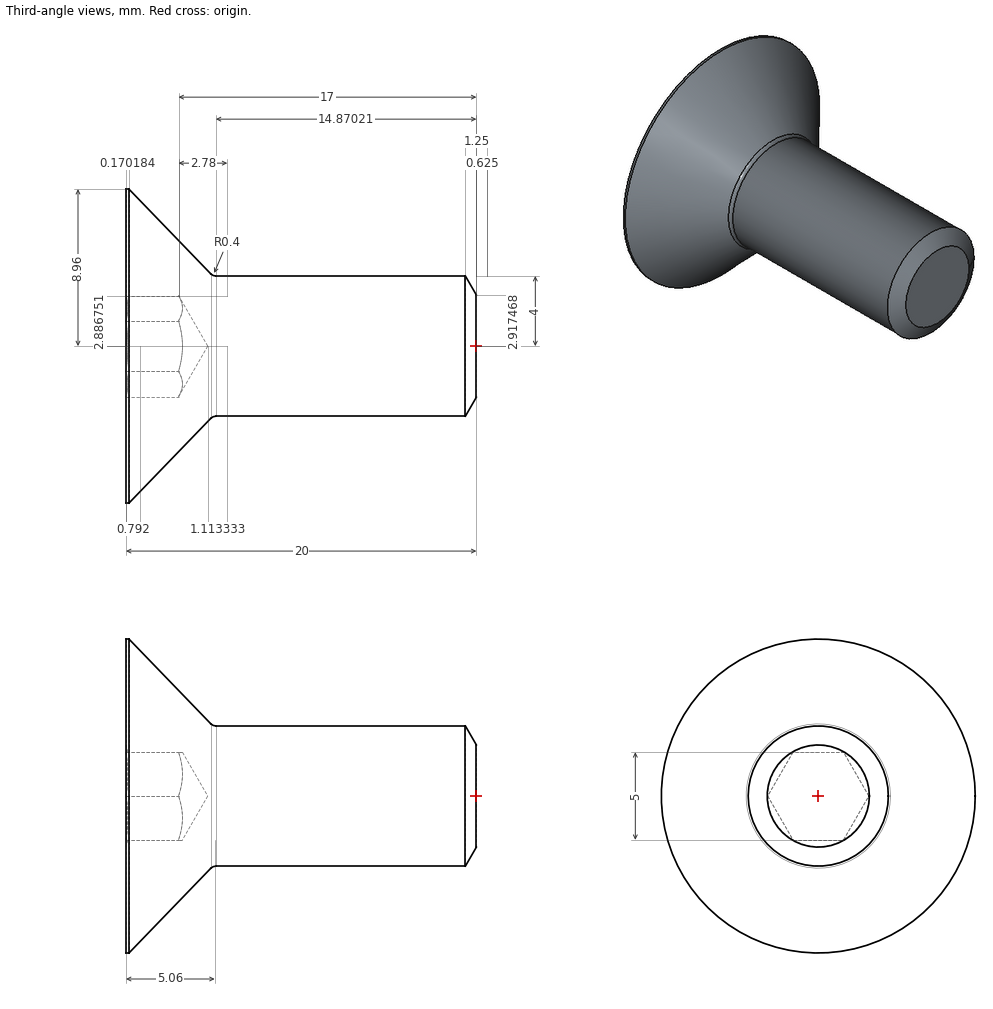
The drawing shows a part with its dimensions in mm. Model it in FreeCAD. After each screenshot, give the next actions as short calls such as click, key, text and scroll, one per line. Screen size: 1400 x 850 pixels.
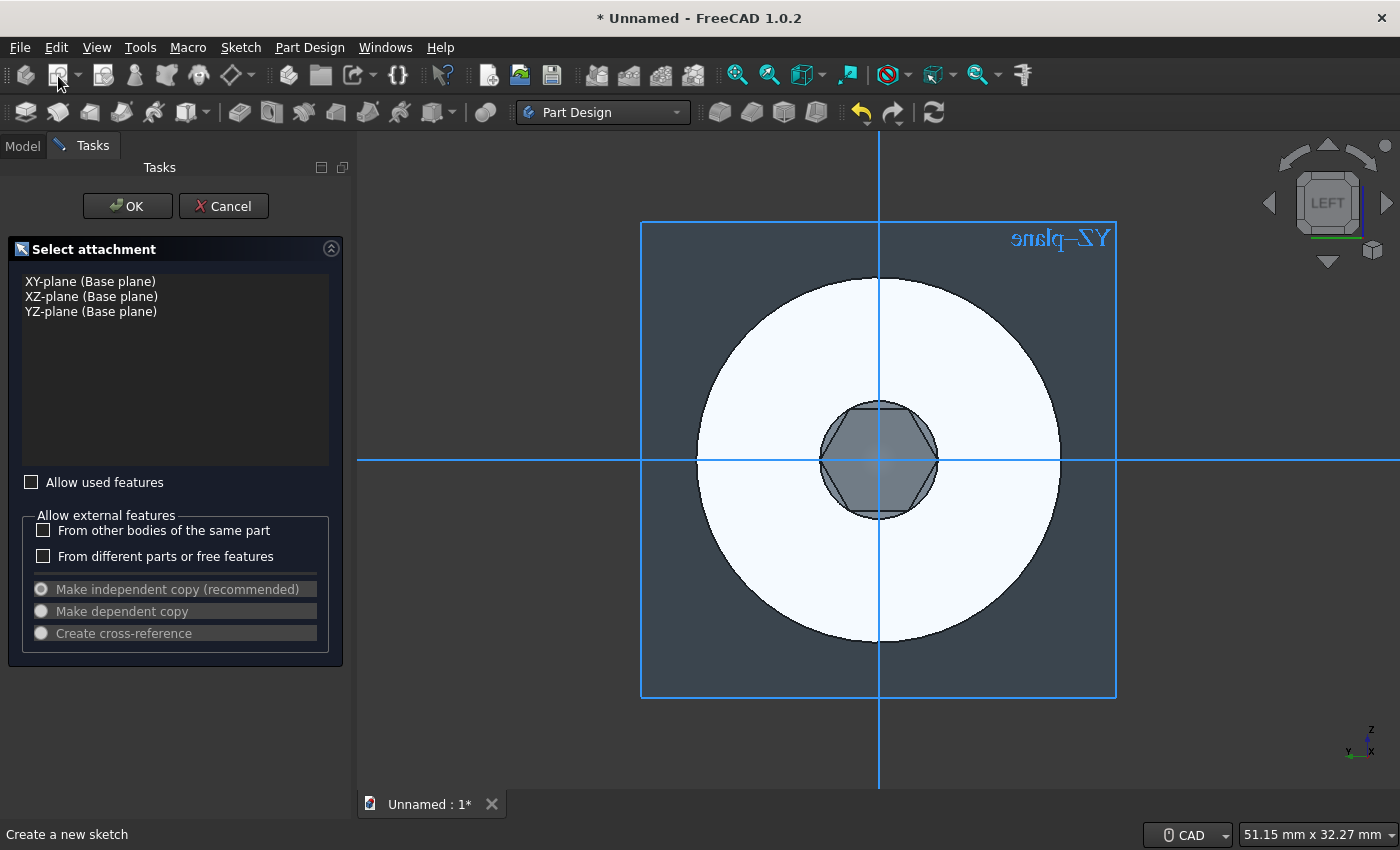
click(82, 282)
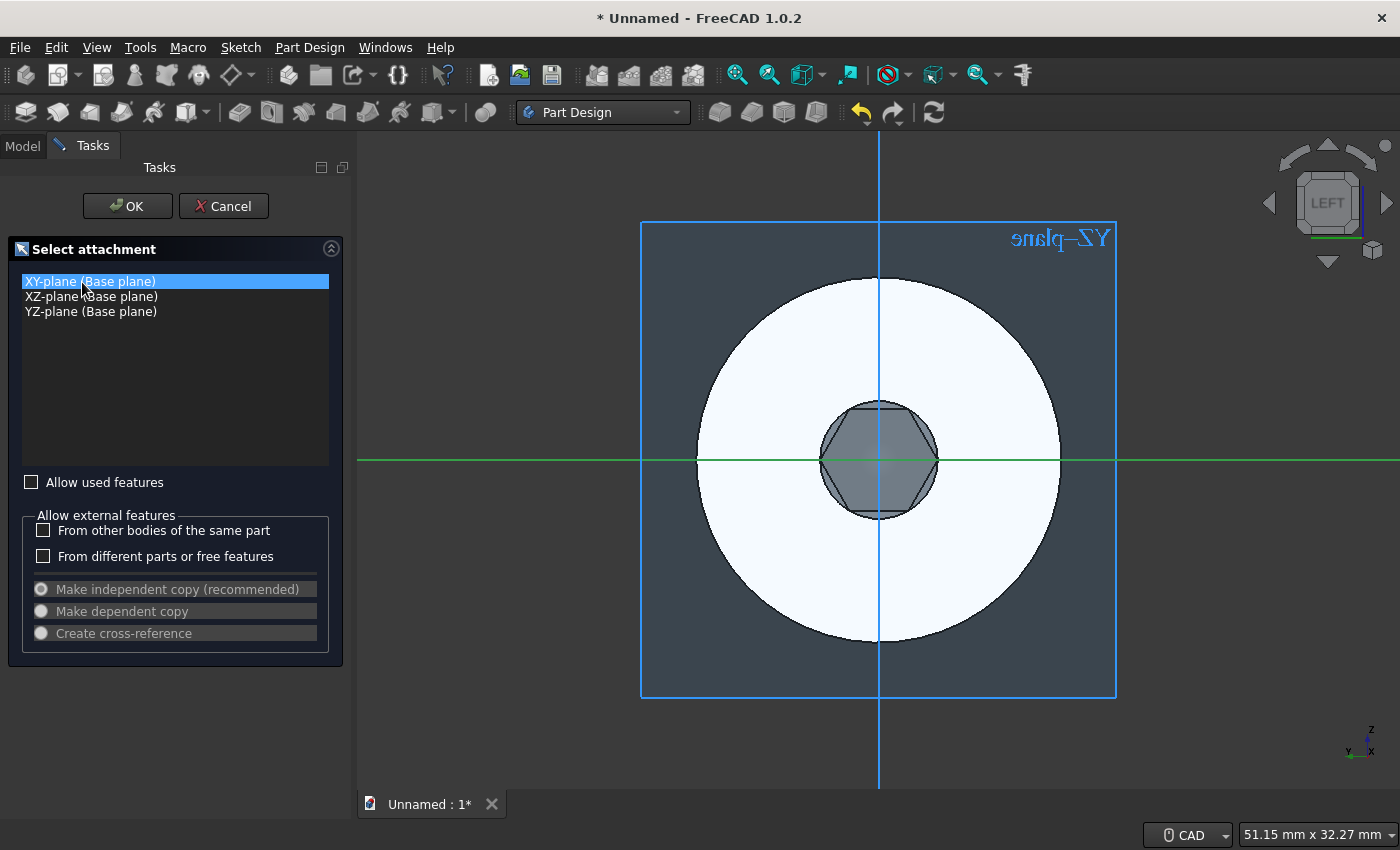
click(128, 206)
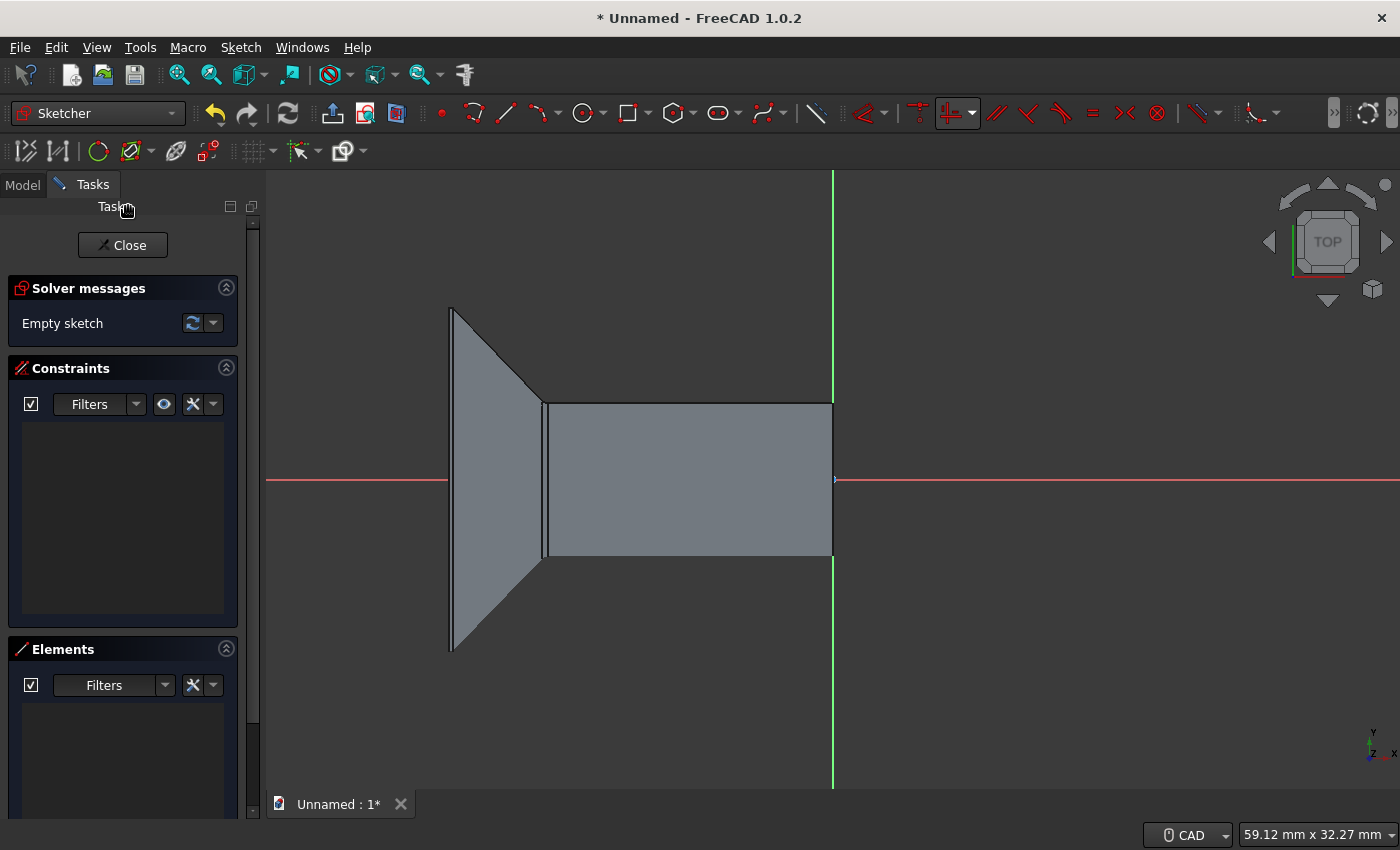
click(398, 114)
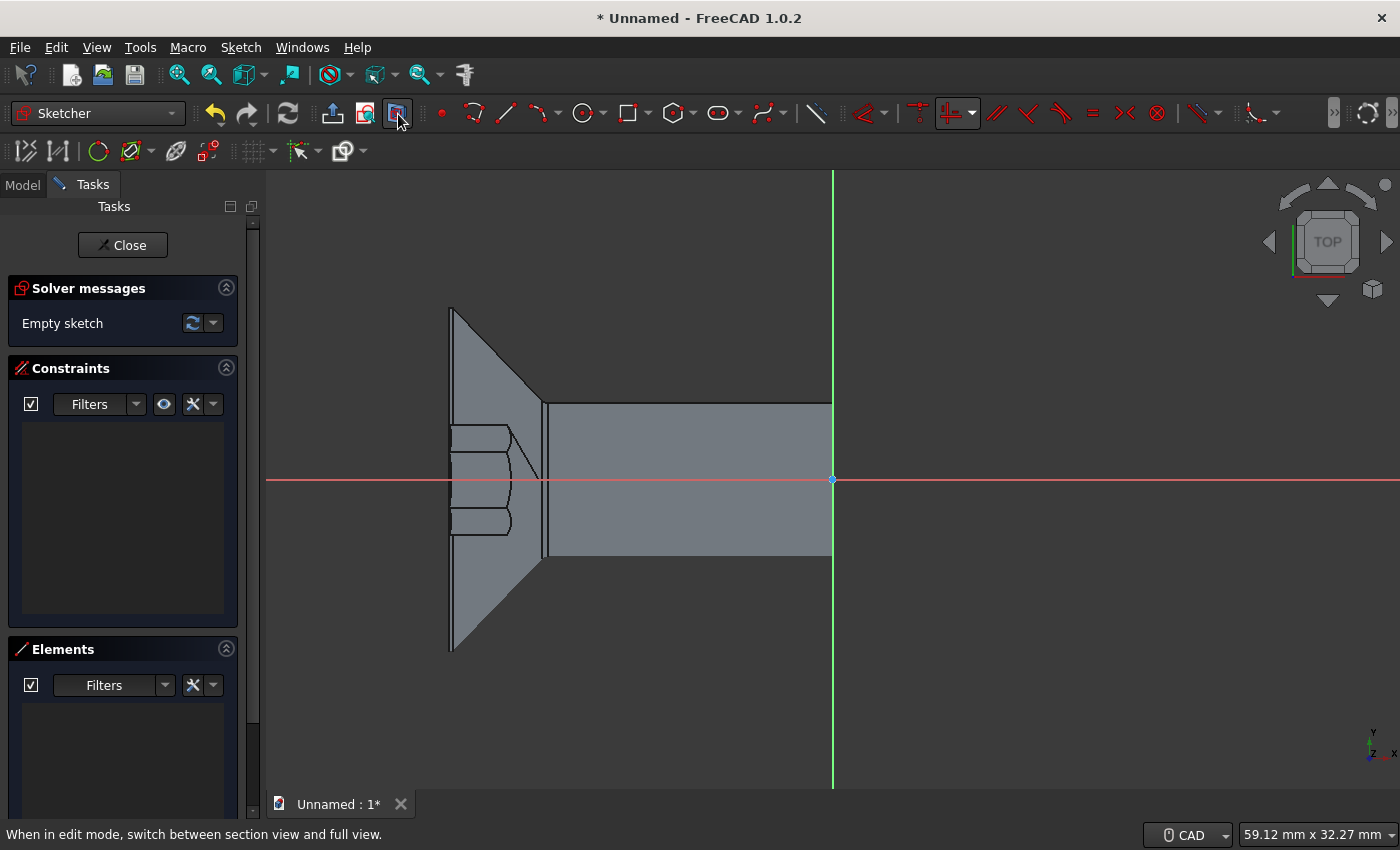
scroll(837, 410, up, 15)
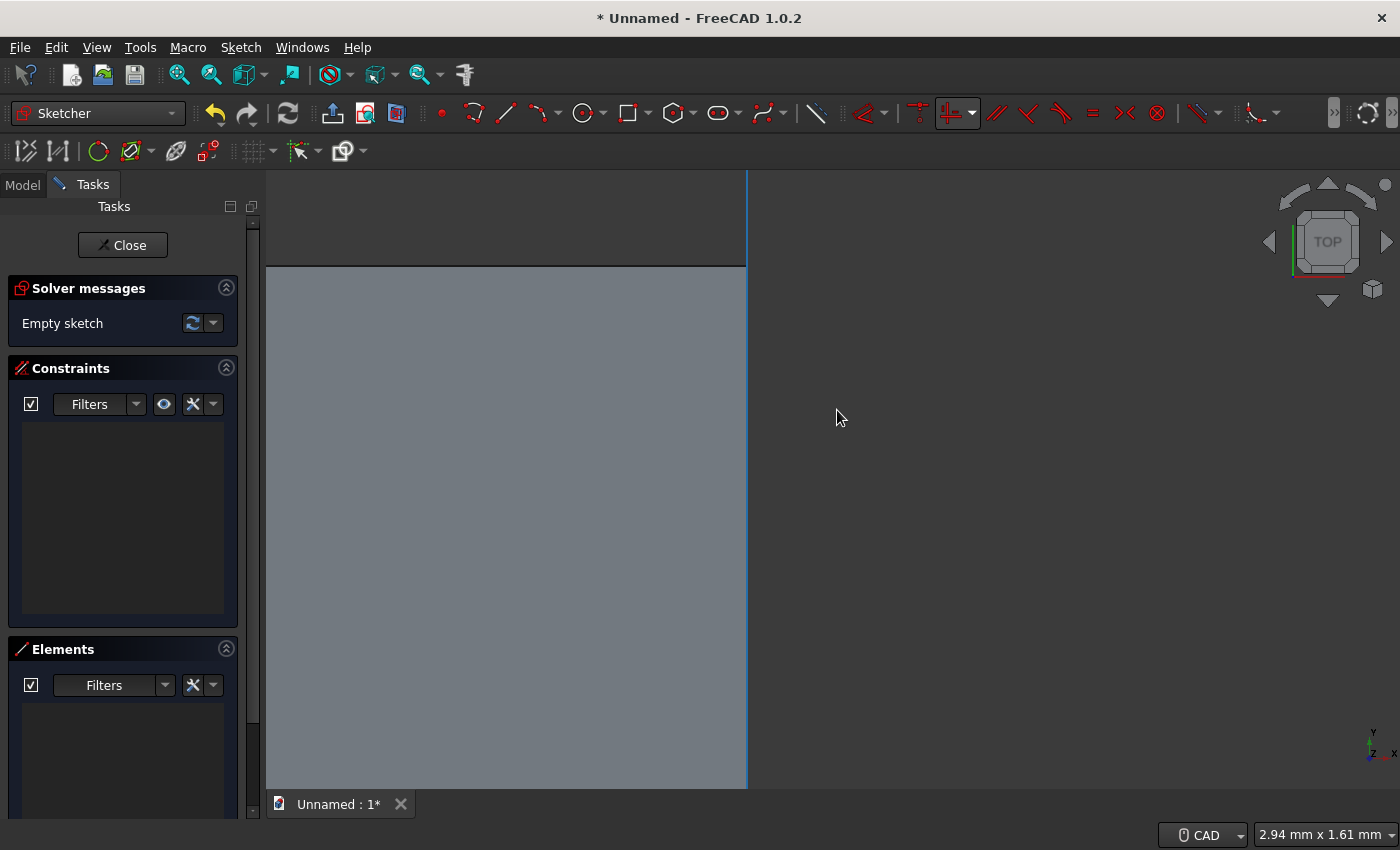
click(474, 114)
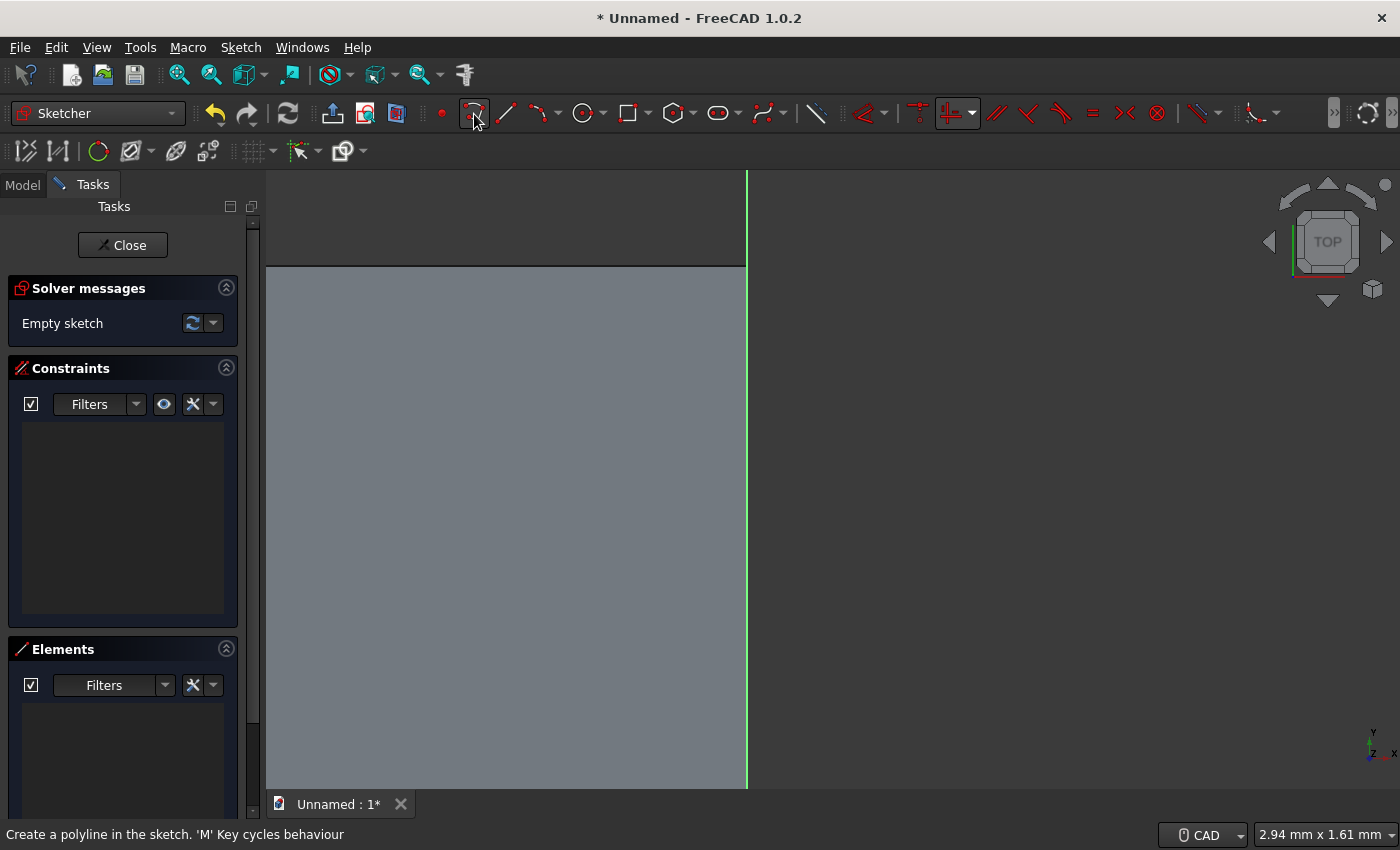
click(747, 683)
click(988, 266)
click(506, 266)
click(747, 684)
key(Escape)
key(Escape)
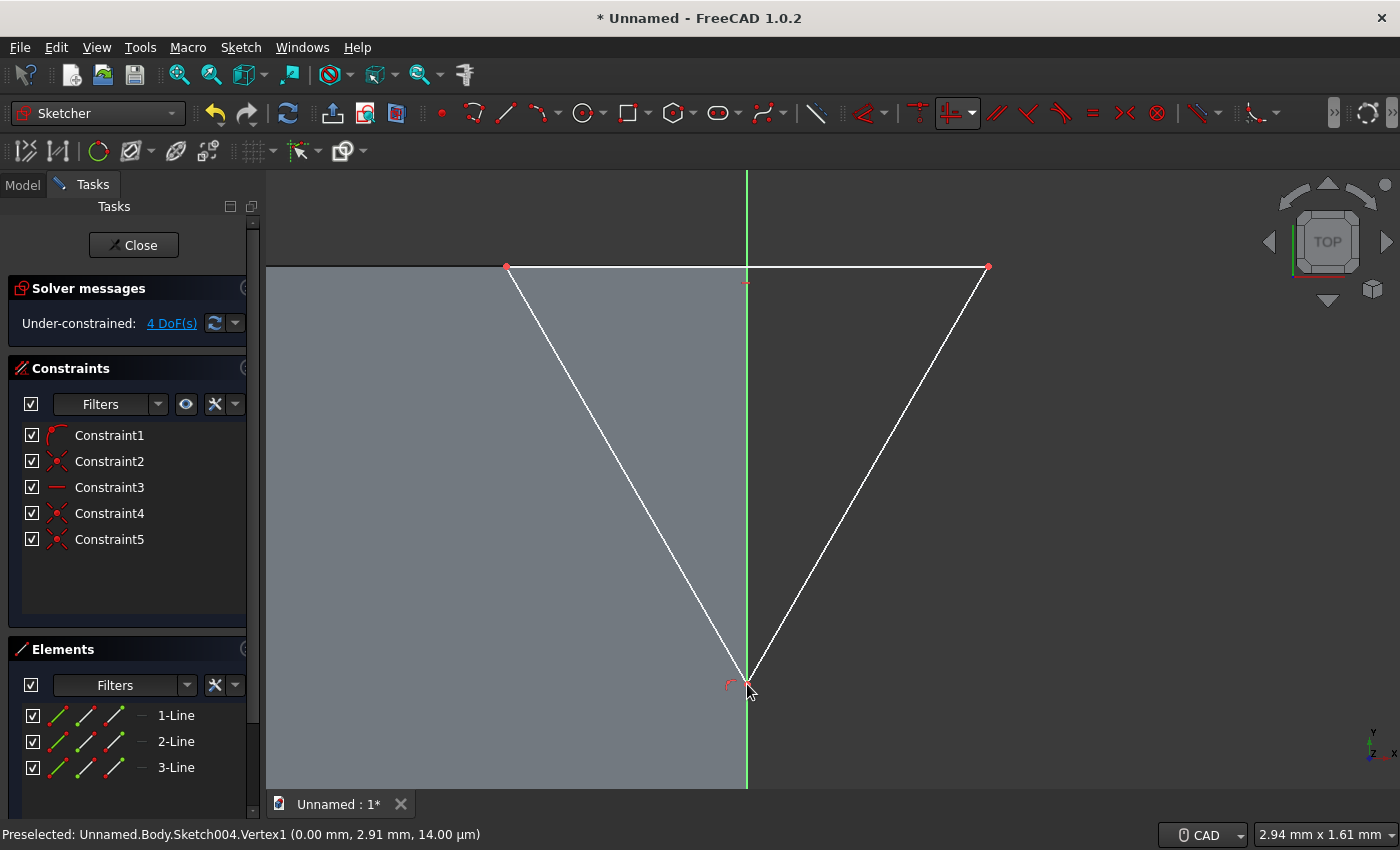
click(864, 114)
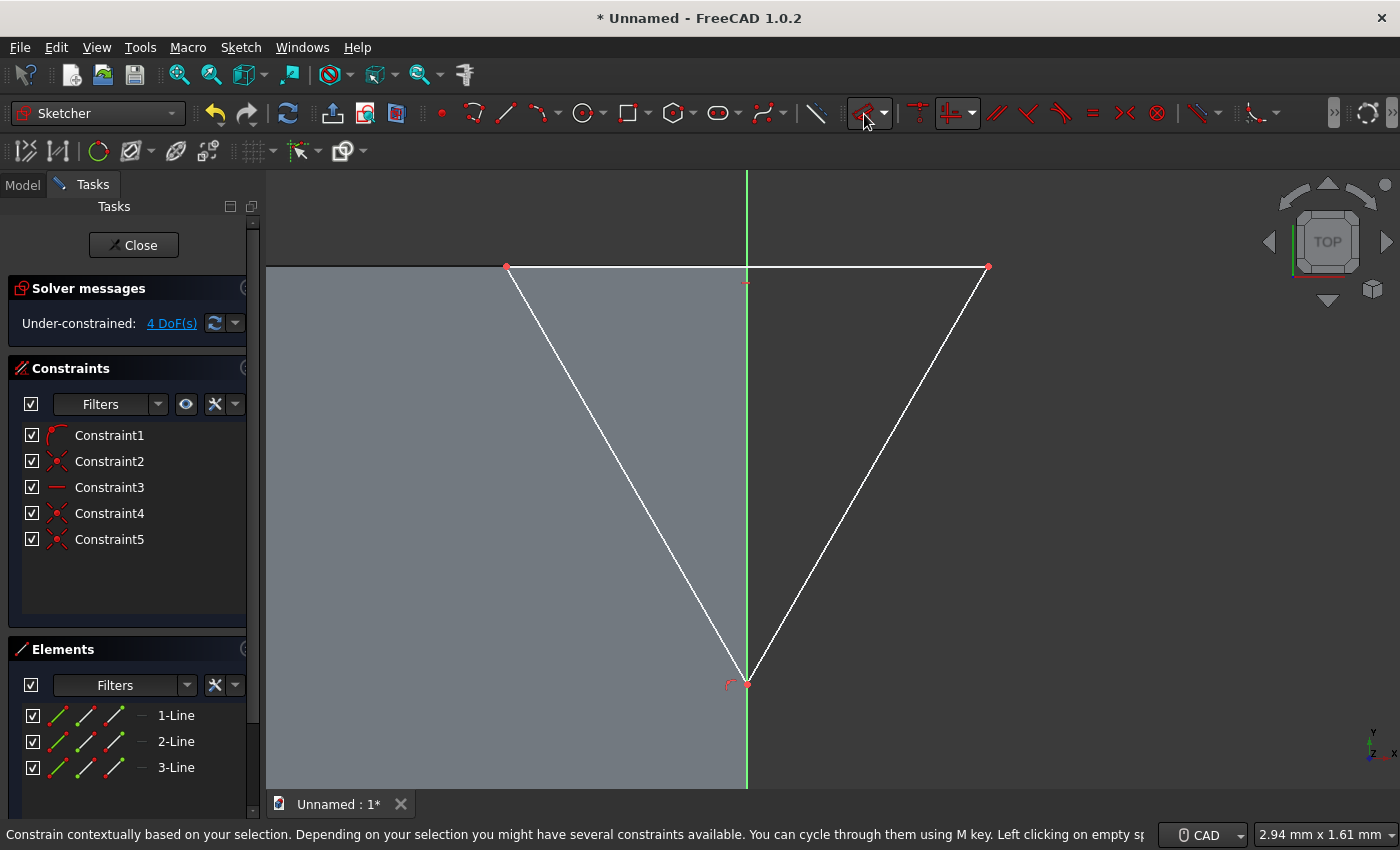
click(988, 267)
click(1022, 514)